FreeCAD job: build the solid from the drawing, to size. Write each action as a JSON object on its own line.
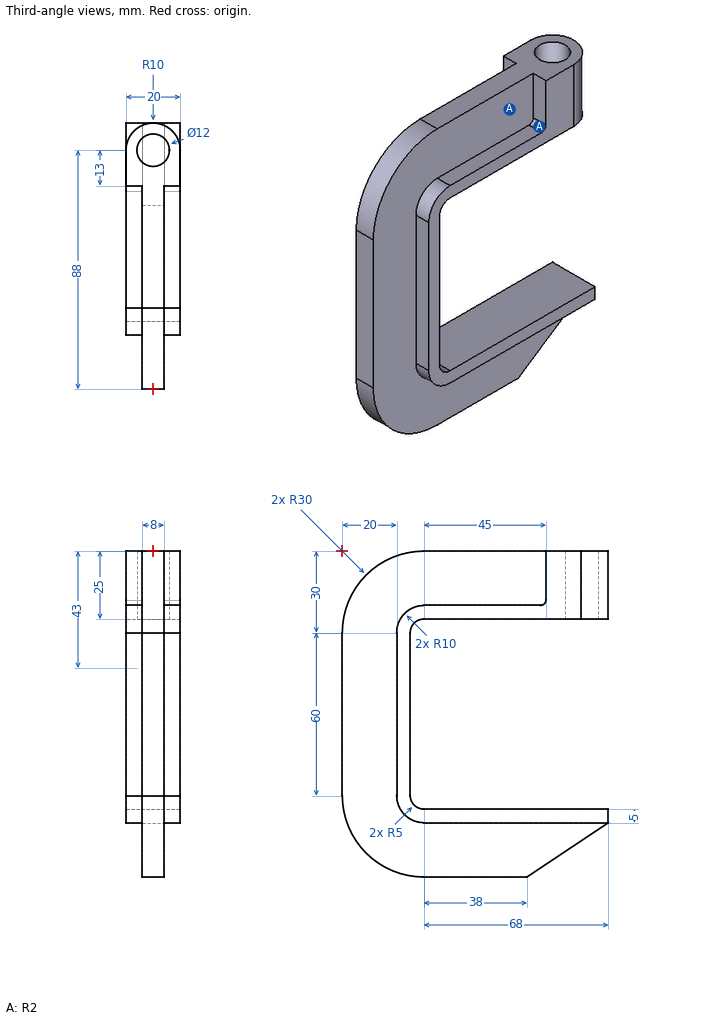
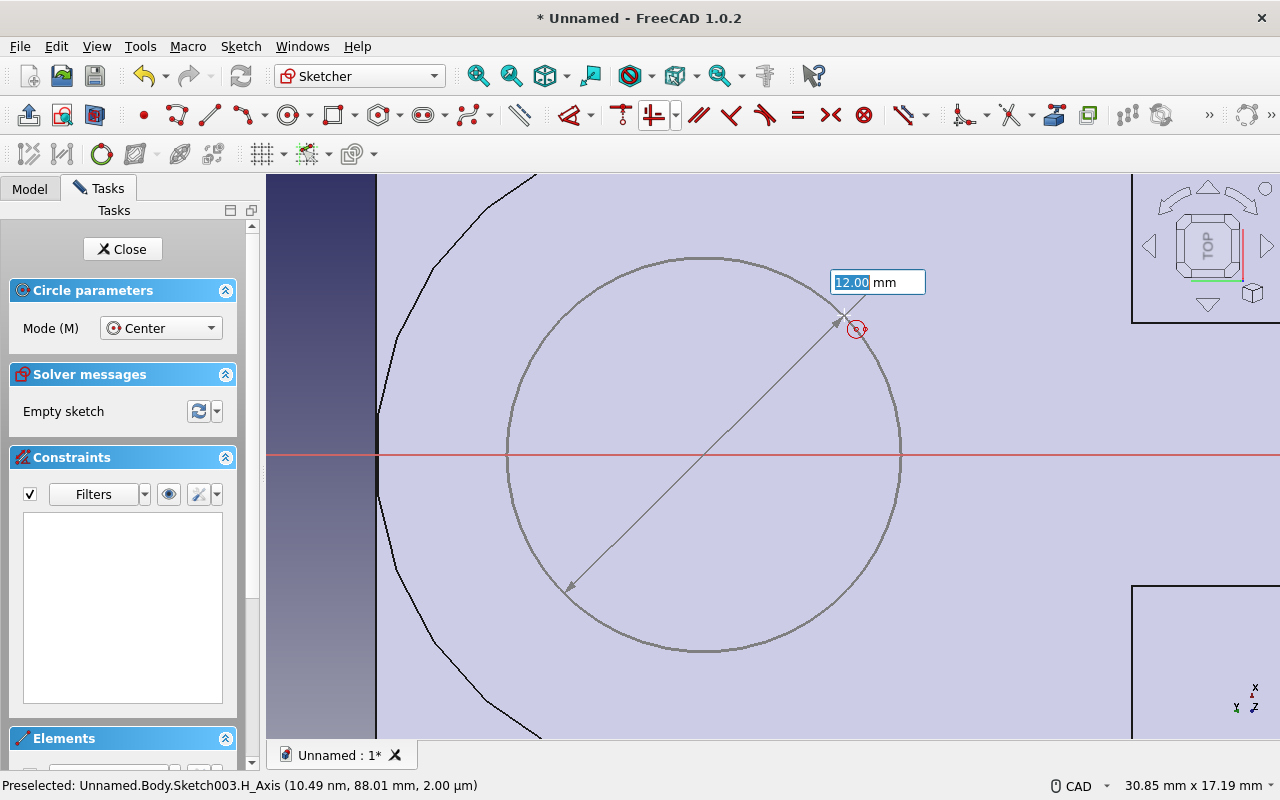
{"action": "type", "text": "12"}
{"action": "key", "text": "Return"}
{"action": "key", "text": "Escape"}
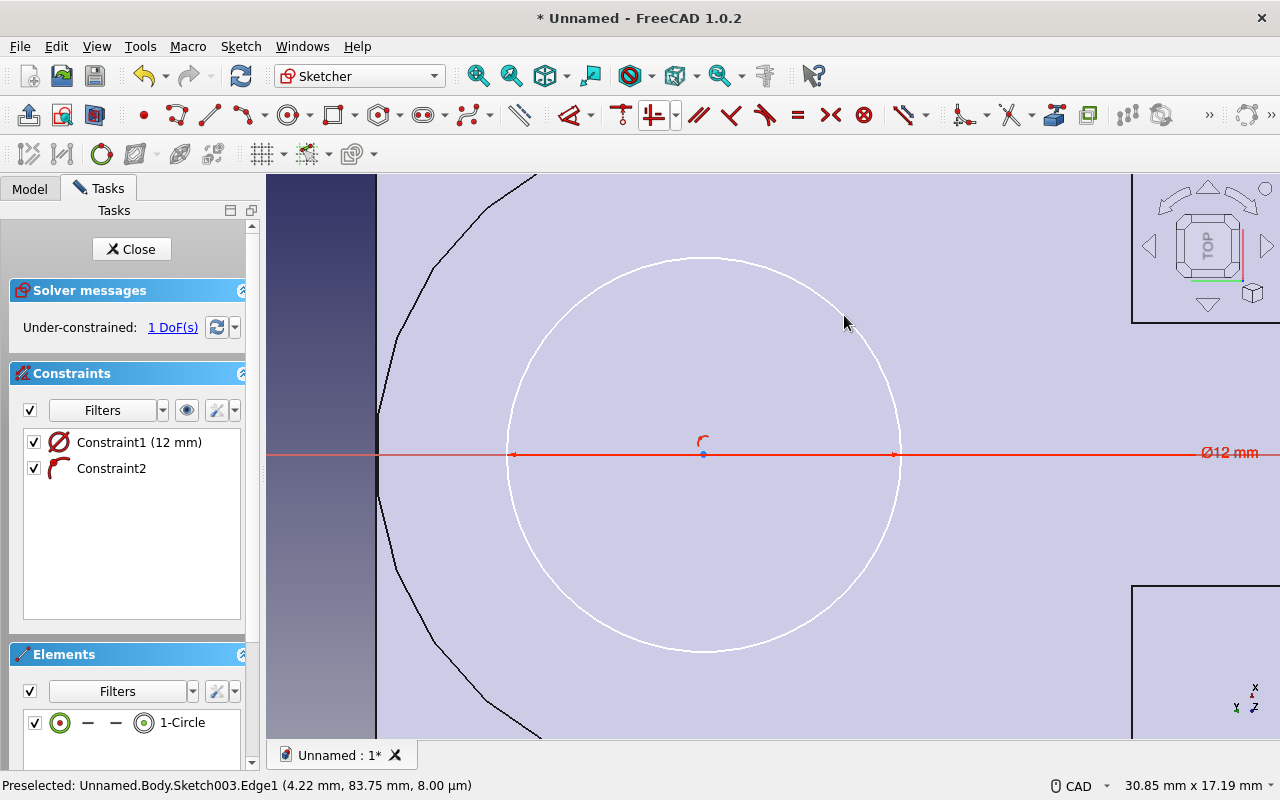
{"action": "key", "text": "d"}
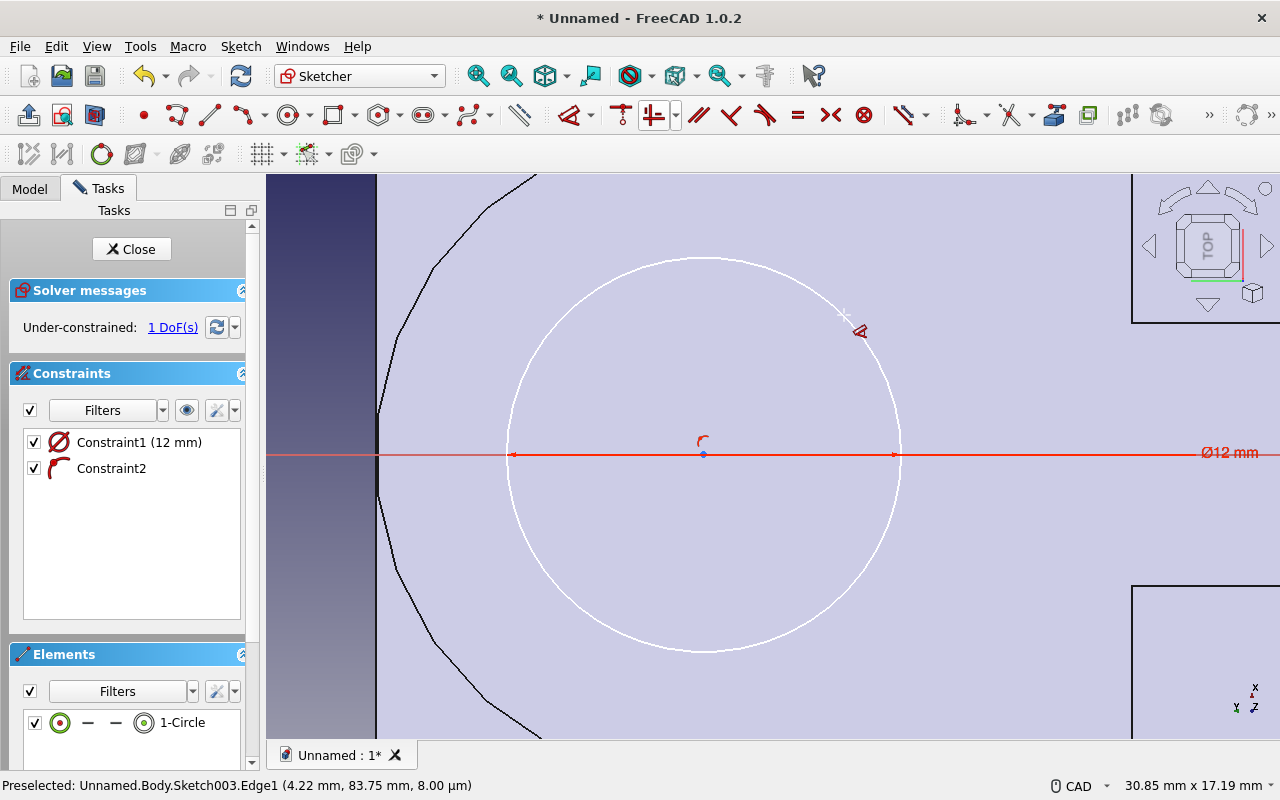
{"action": "left_click", "coordinate": [704, 455]}
{"action": "left_click", "coordinate": [815, 421]}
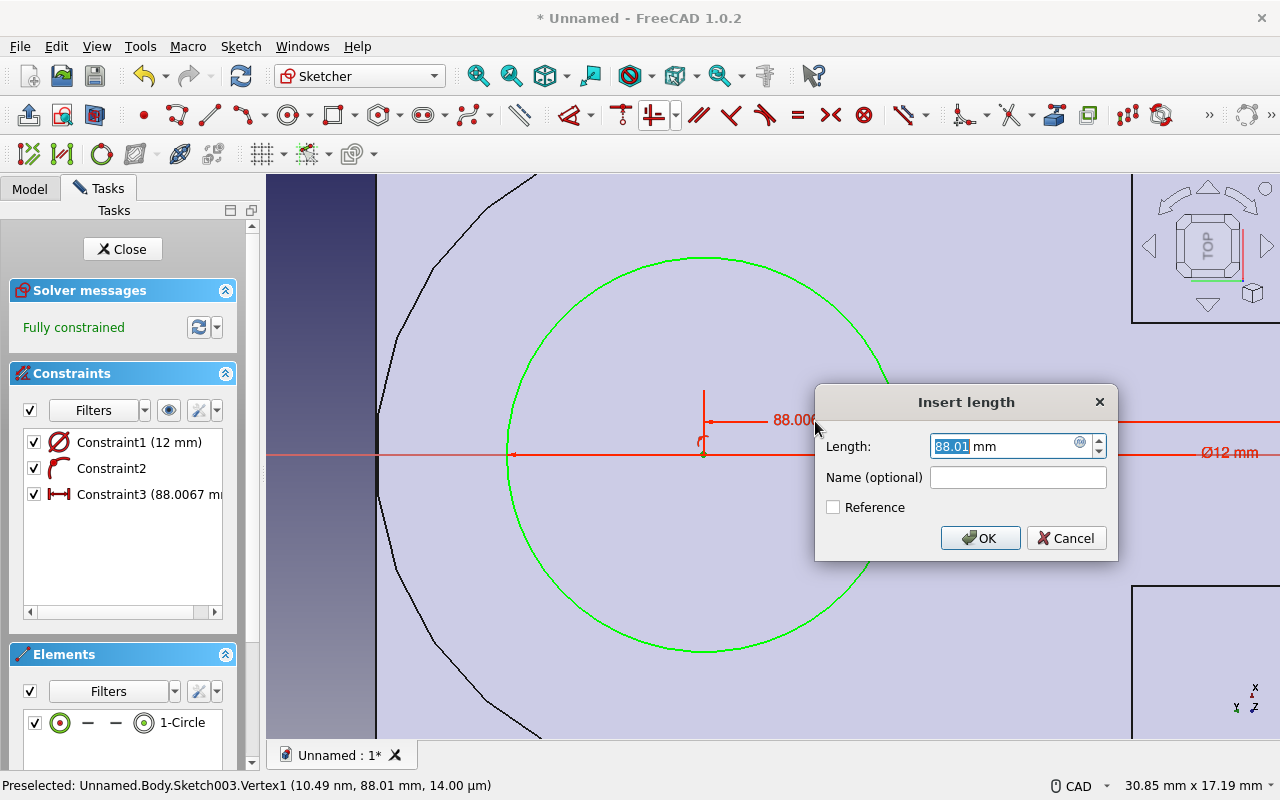
{"action": "type", "text": "88"}
{"action": "key", "text": "Return"}
{"action": "key", "text": "Escape"}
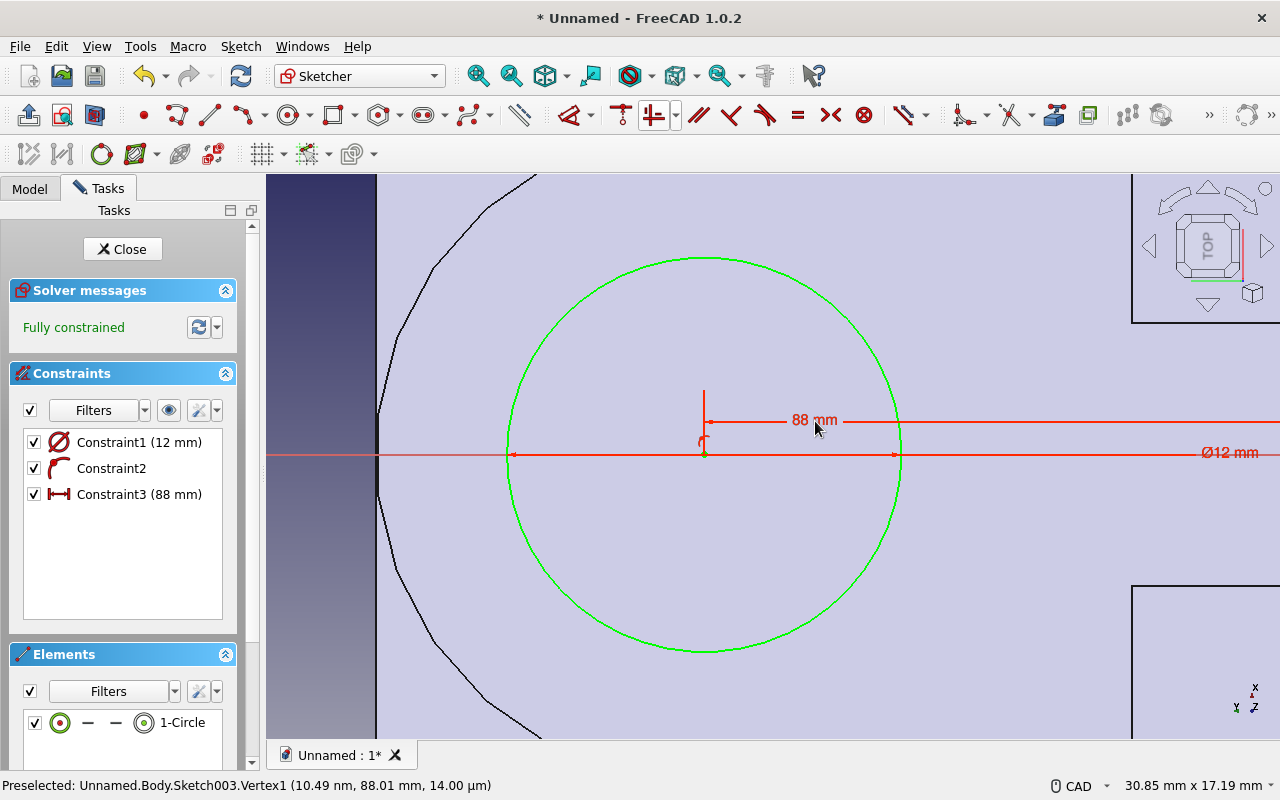
{"action": "left_click", "coordinate": [123, 249]}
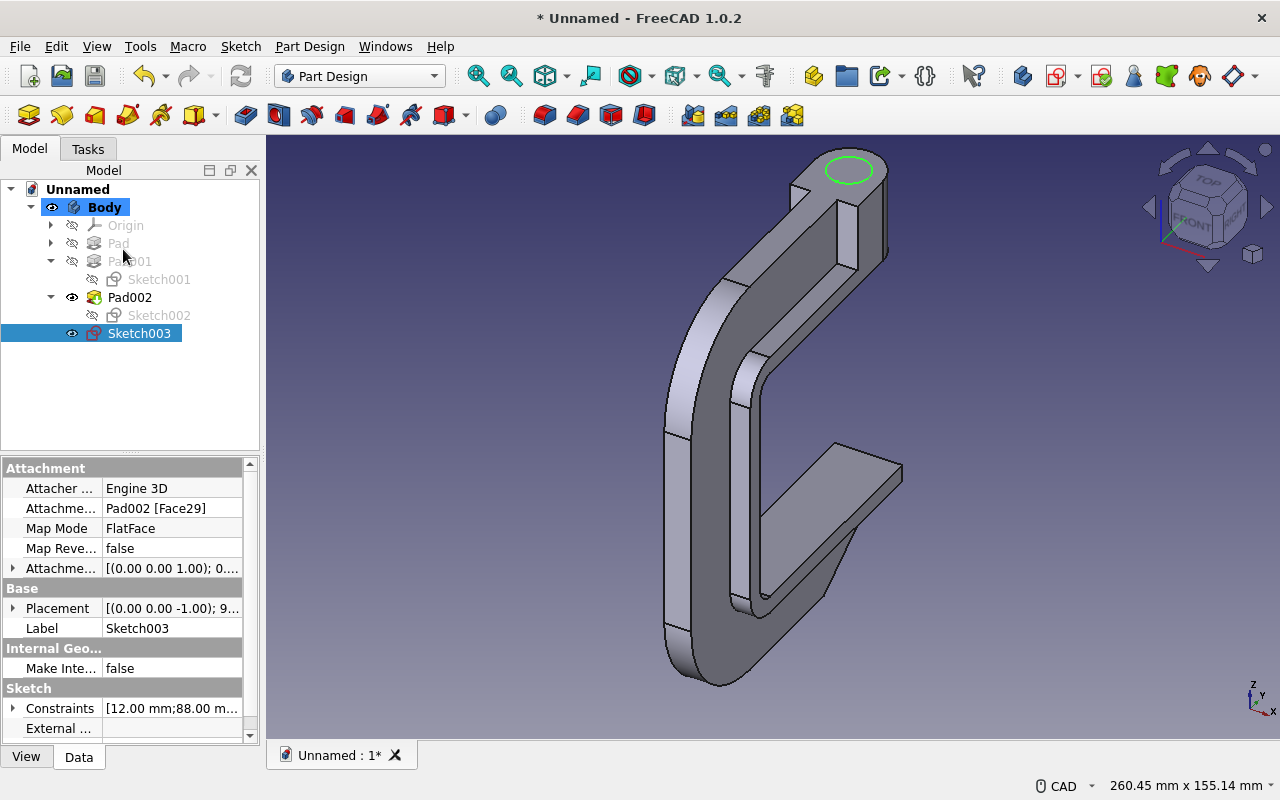
{"action": "left_click", "coordinate": [246, 116]}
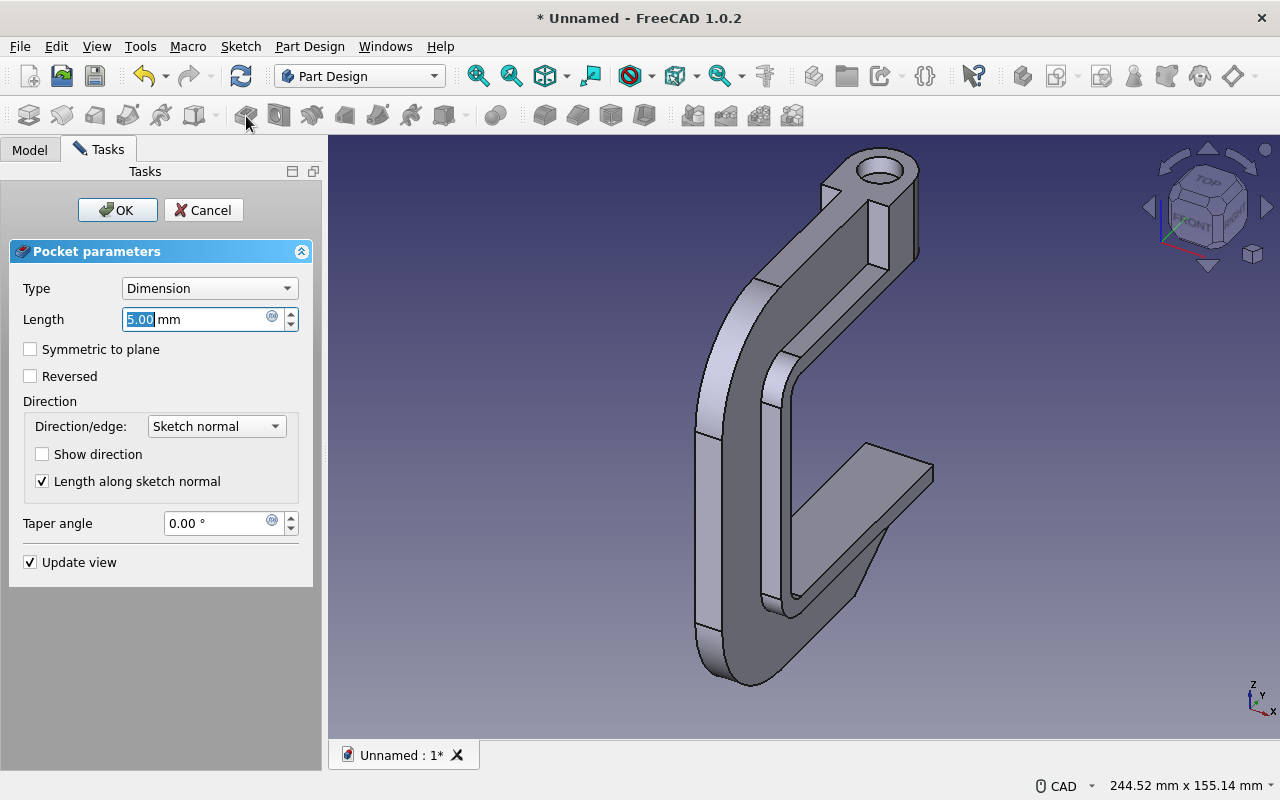
{"action": "type", "text": "43"}
{"action": "key", "text": "Tab"}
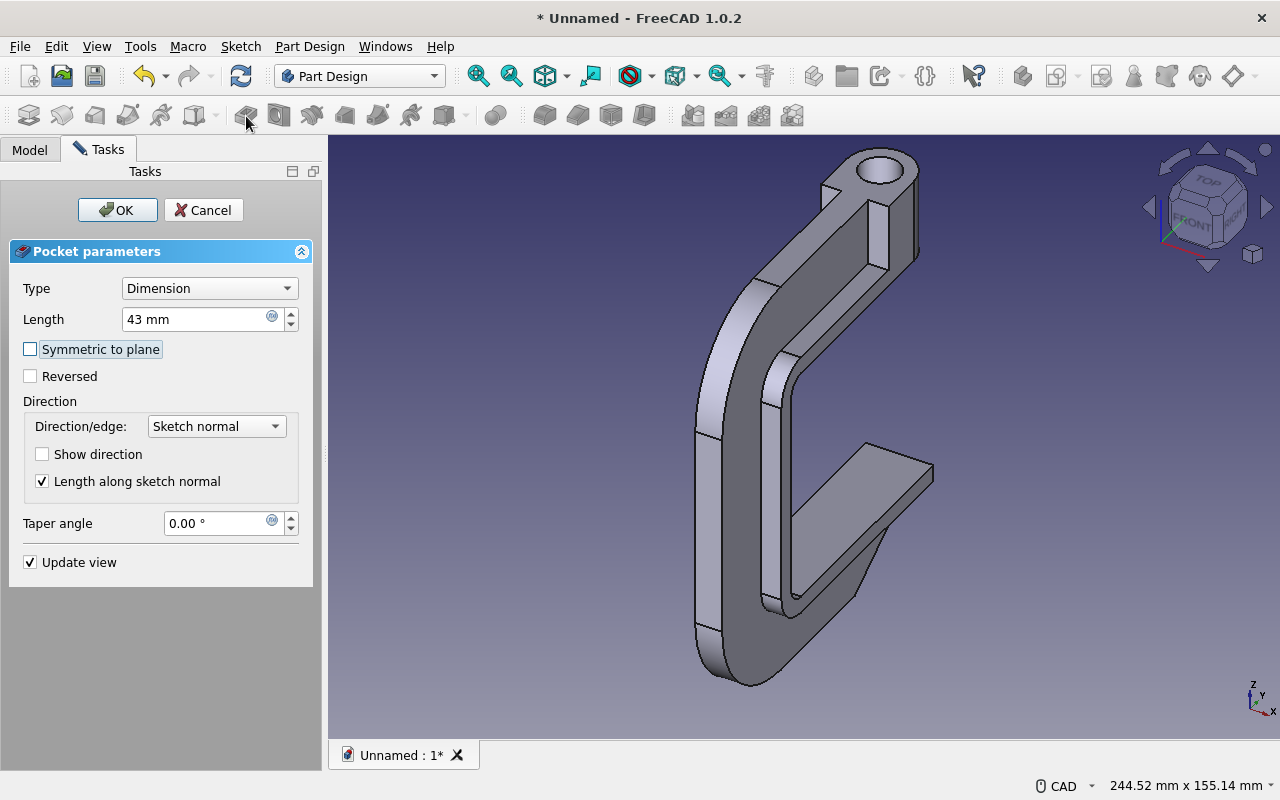
{"action": "left_click", "coordinate": [118, 210]}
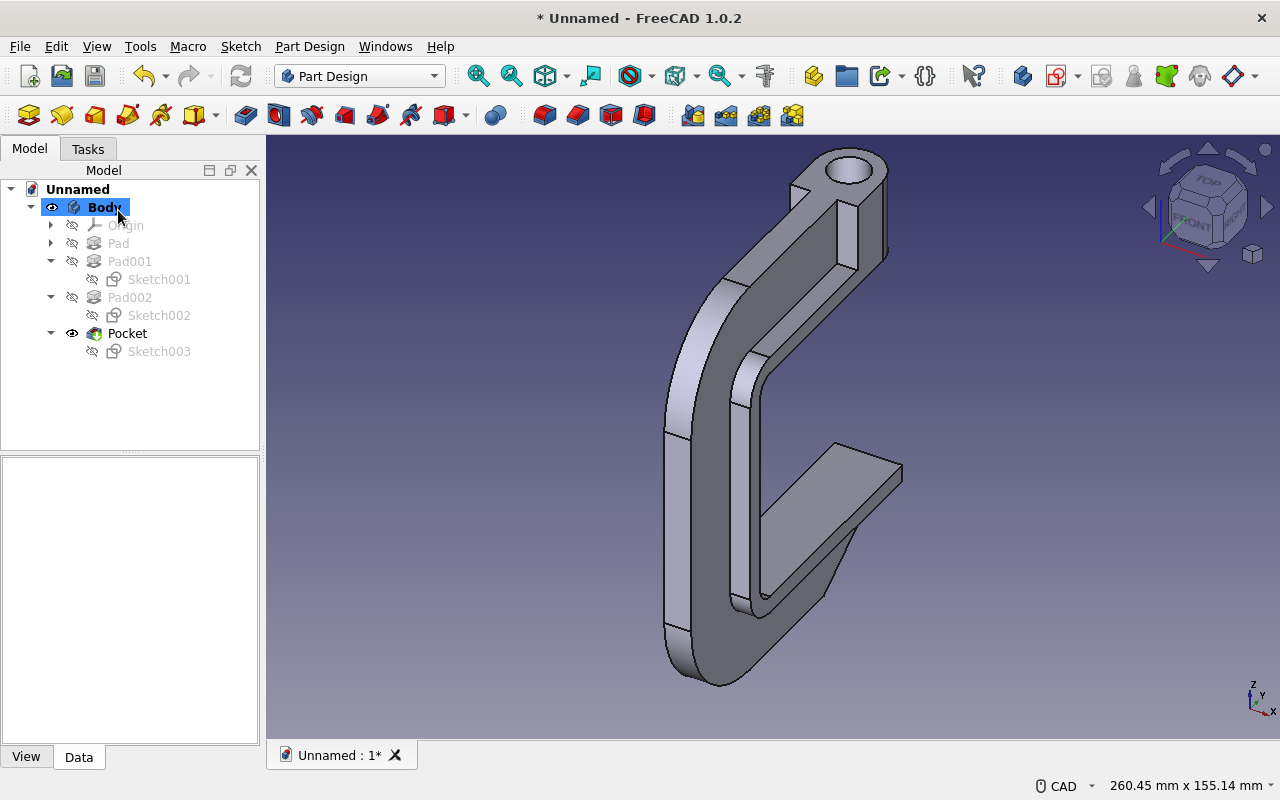
{"action": "key", "text": "0"}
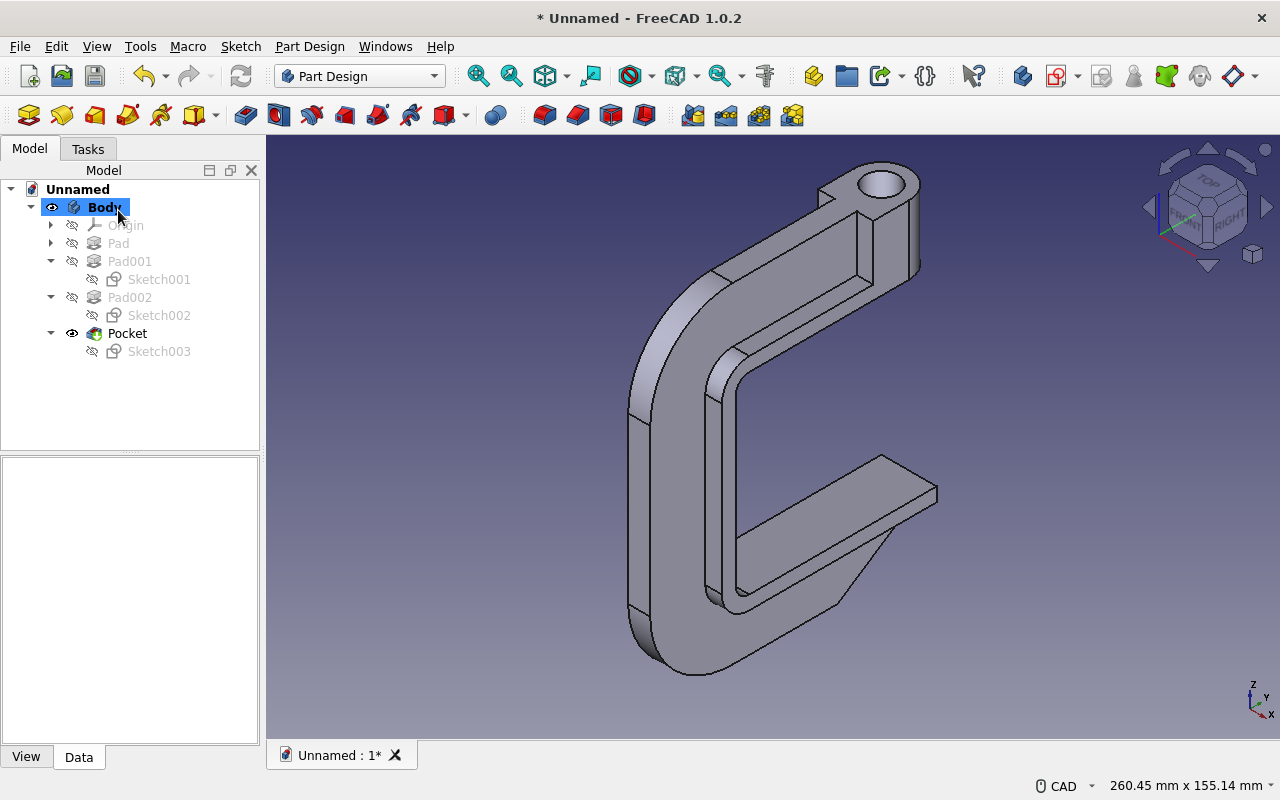
{"action": "key", "text": "2"}